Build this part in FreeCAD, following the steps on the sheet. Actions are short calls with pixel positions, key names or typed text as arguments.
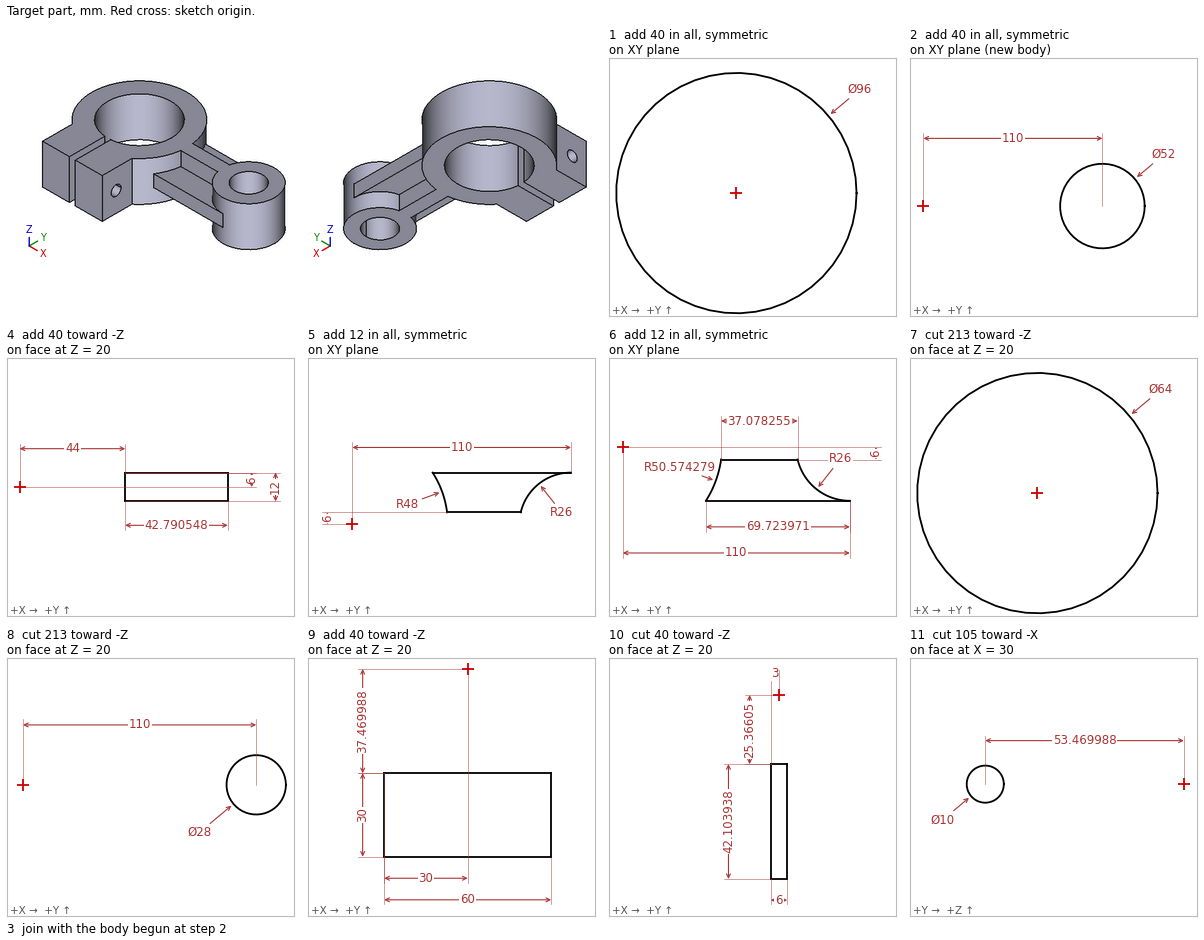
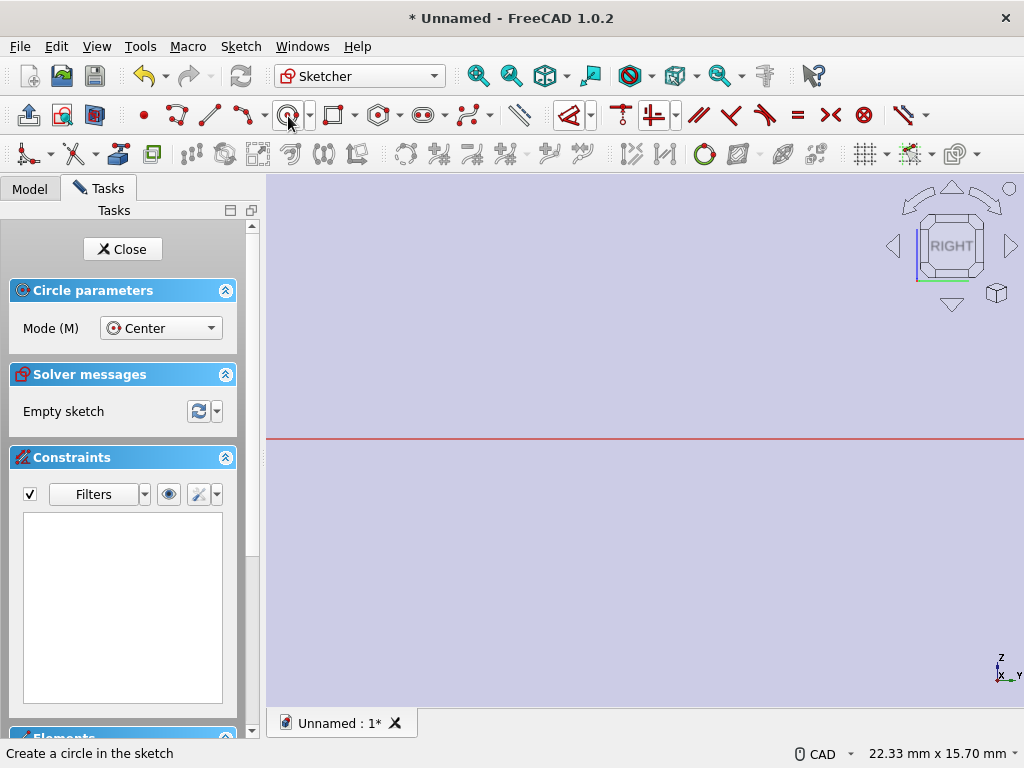
click(570, 439)
click(690, 319)
key(Escape)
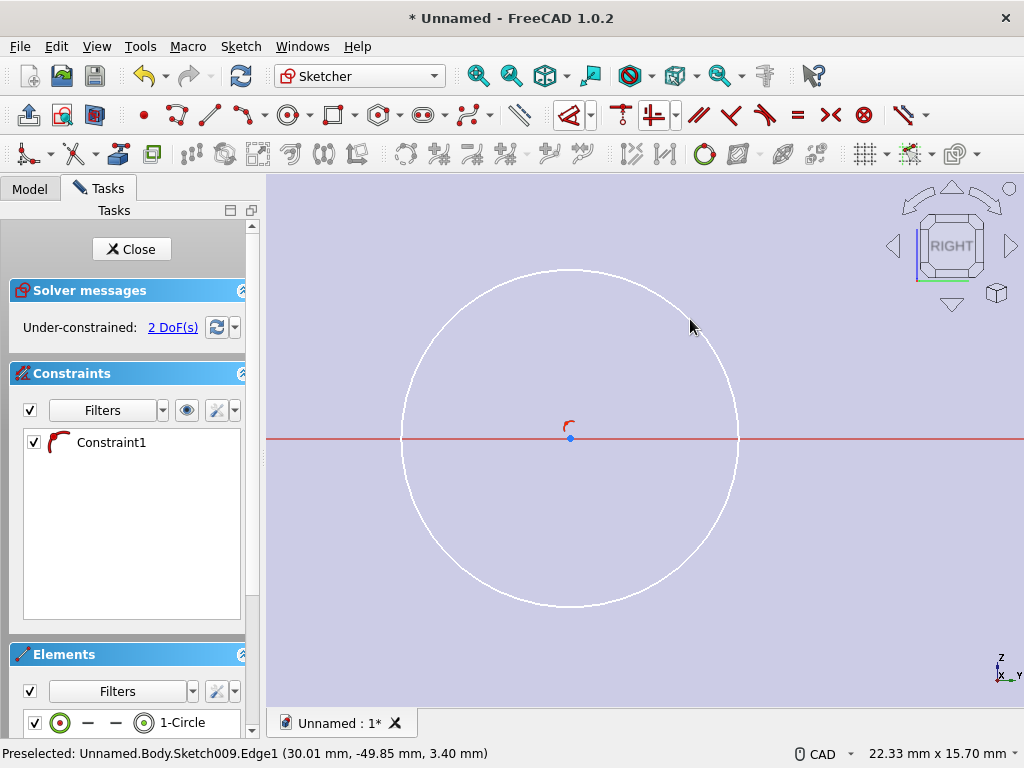
click(689, 319)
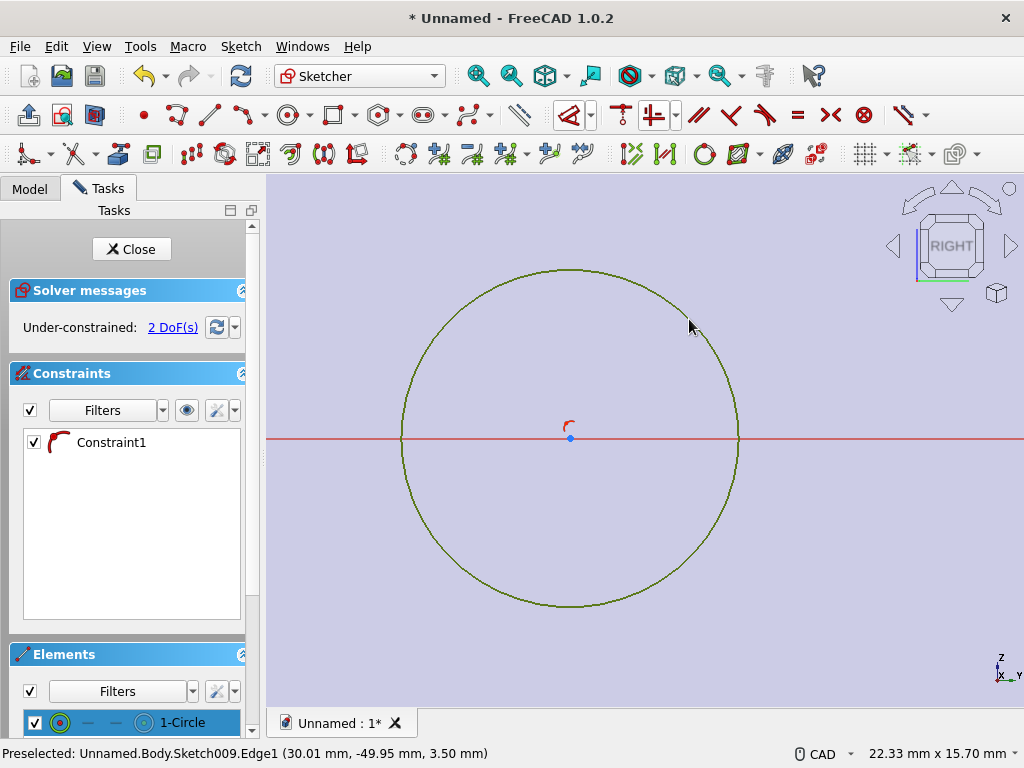
click(590, 116)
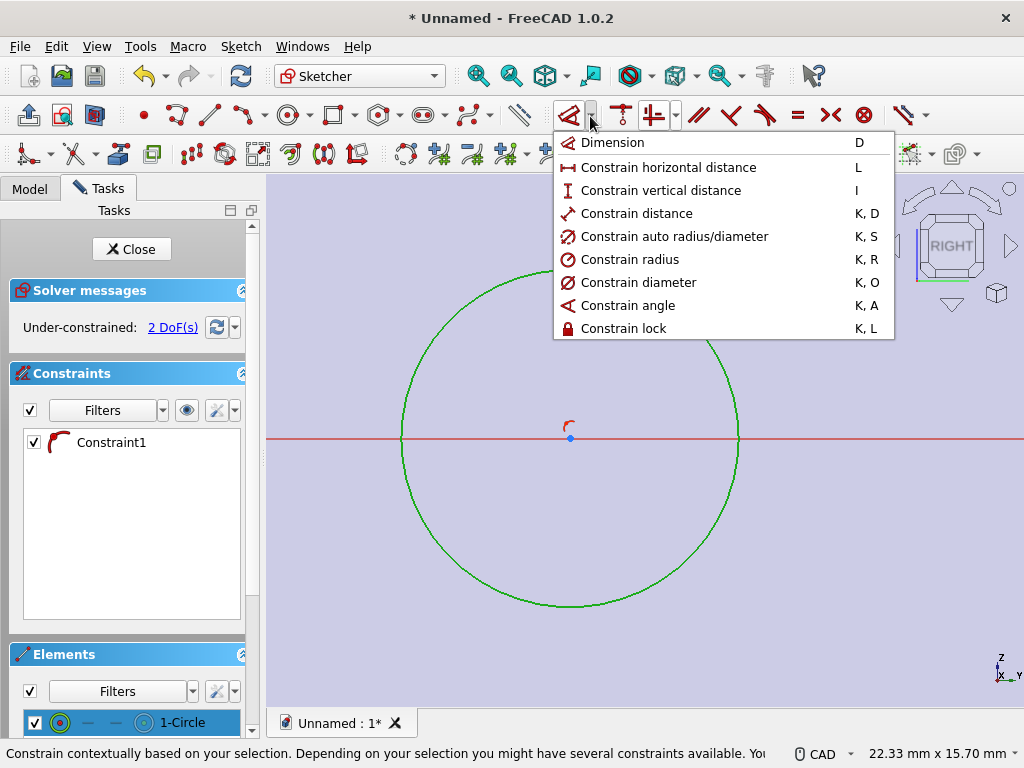
click(724, 282)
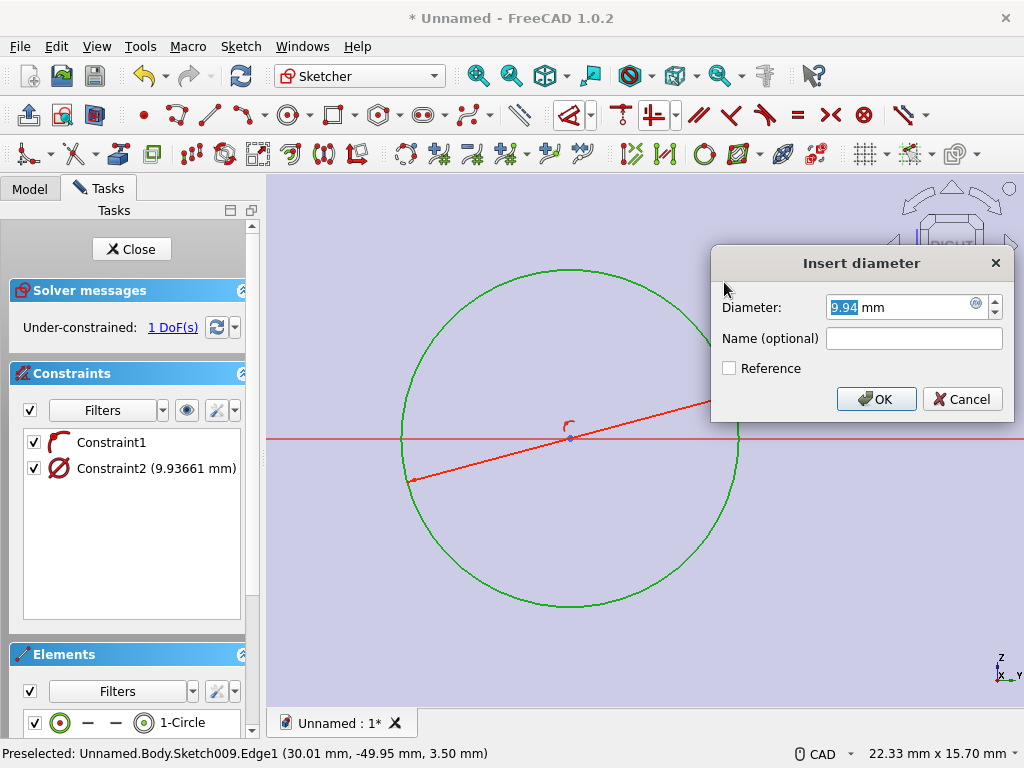
text(10)
key(Return)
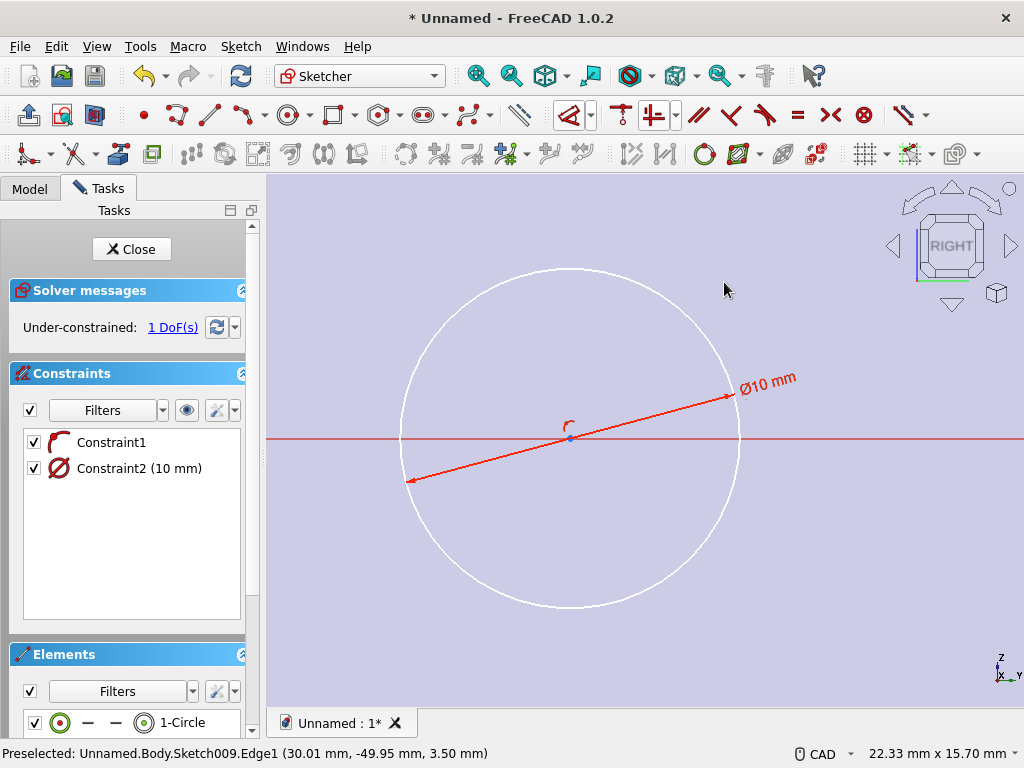
click(570, 439)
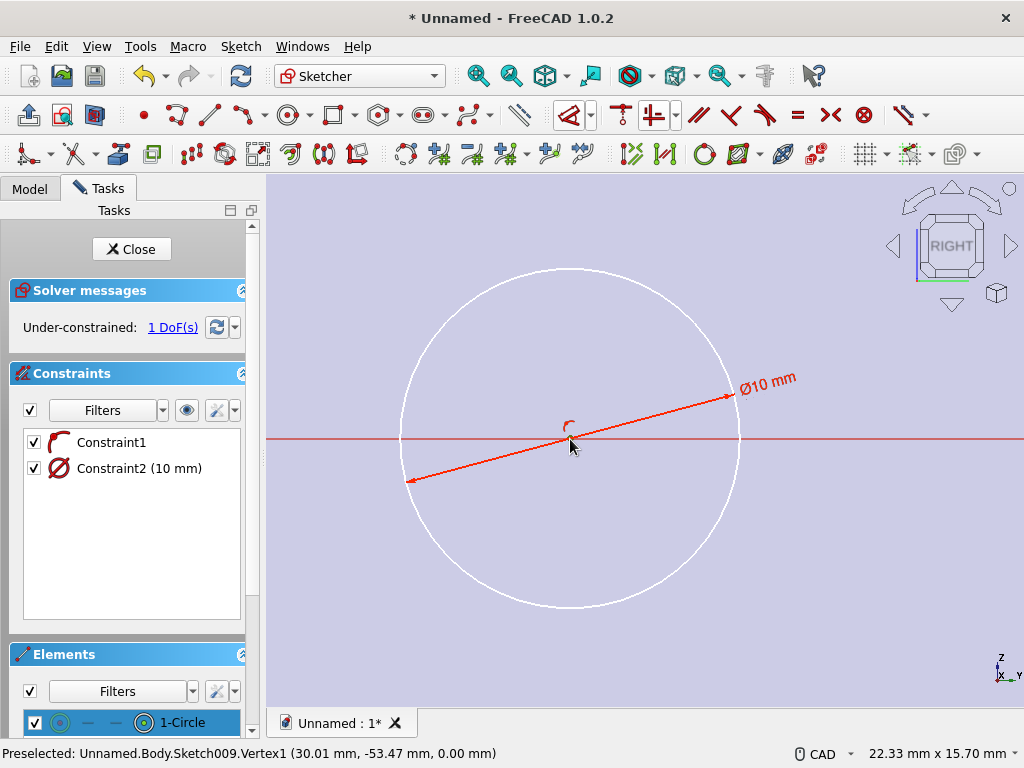
click(590, 116)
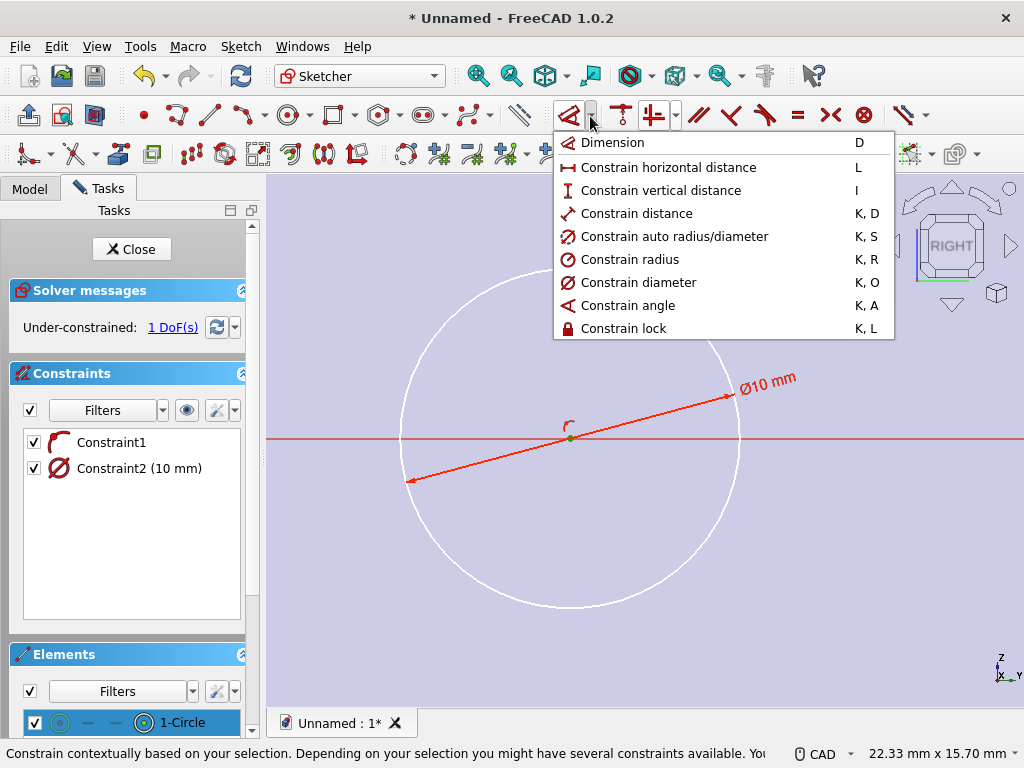
click(724, 168)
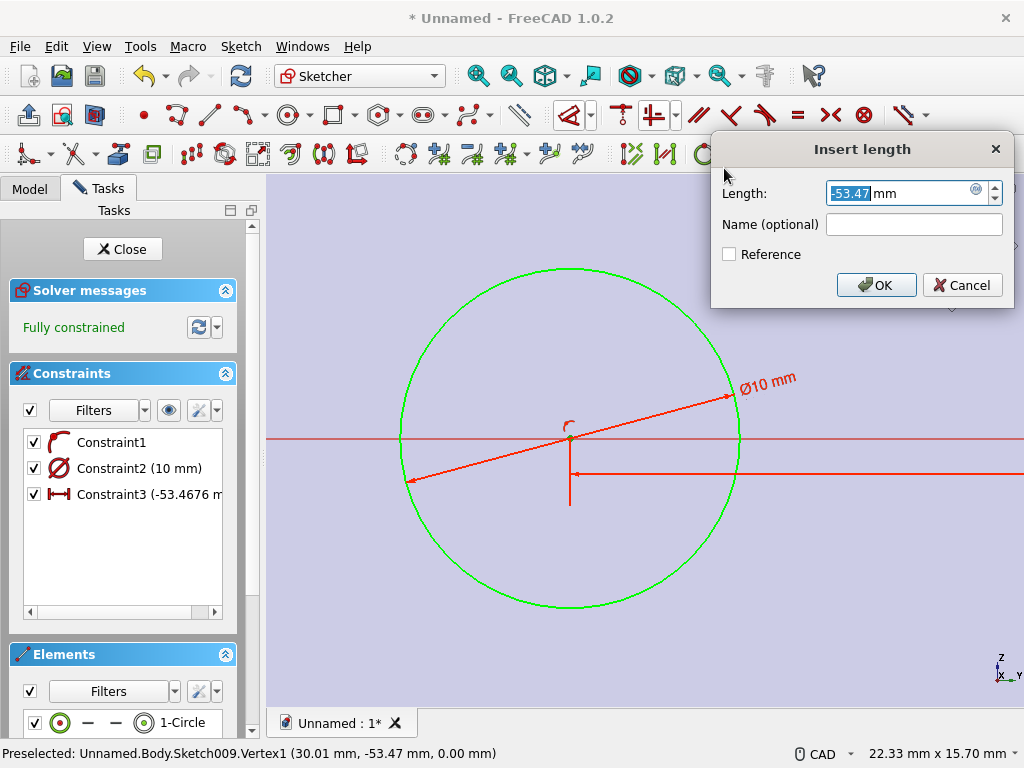
text(-53.469988)
key(Return)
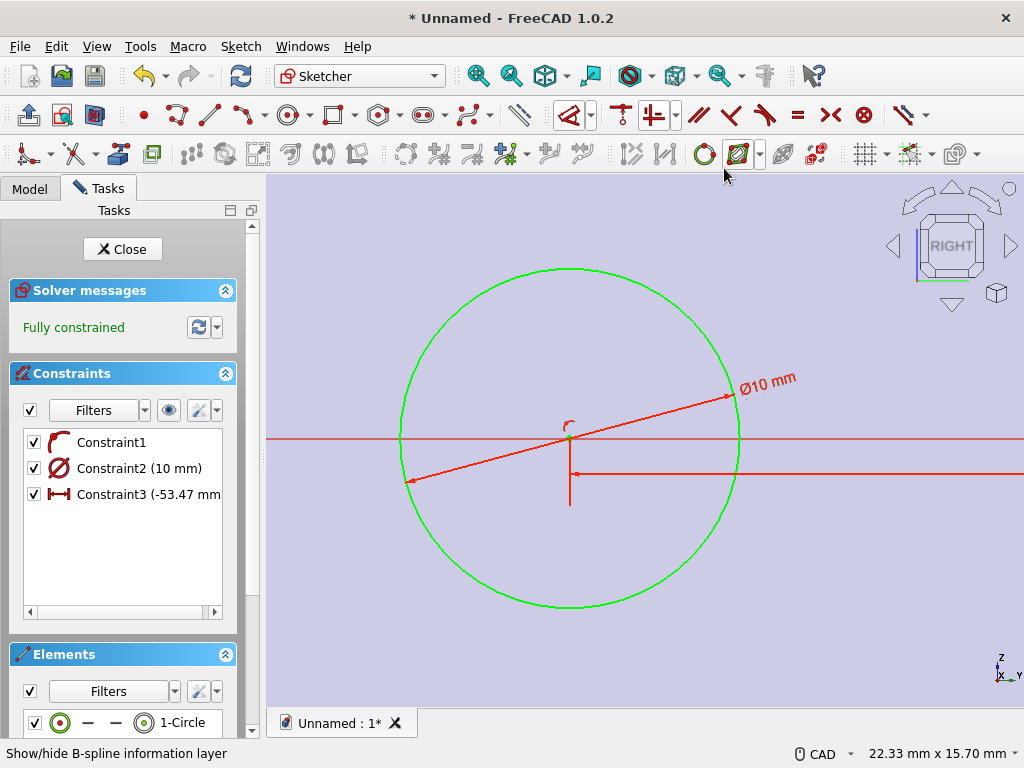
click(123, 249)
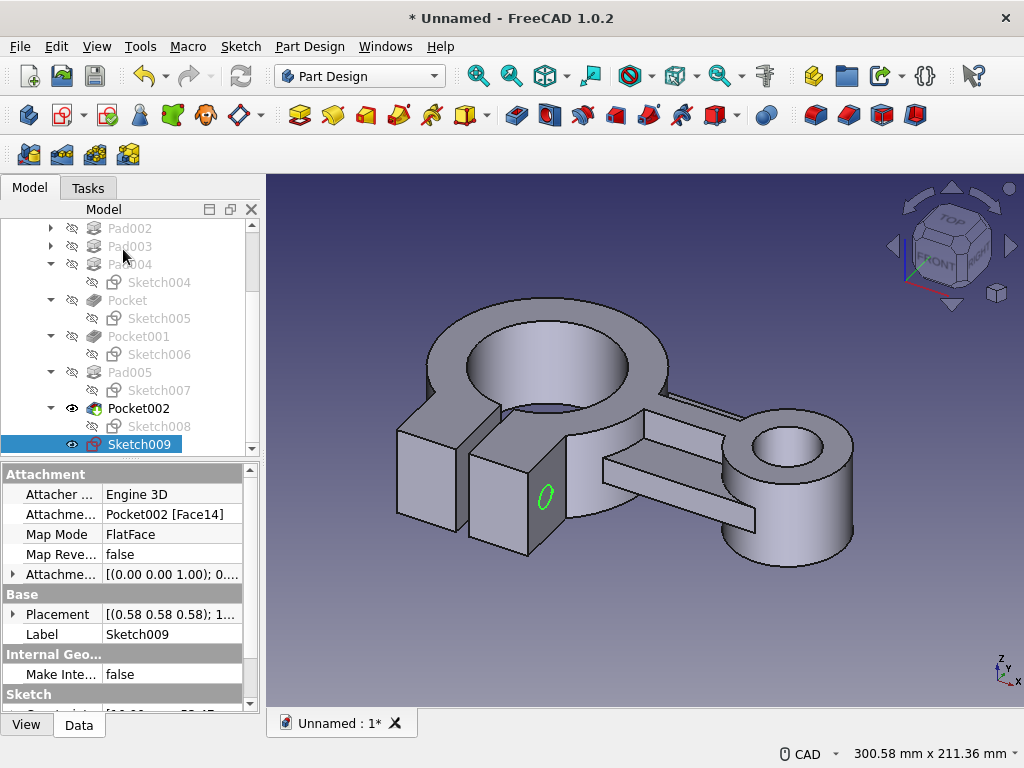
click(517, 116)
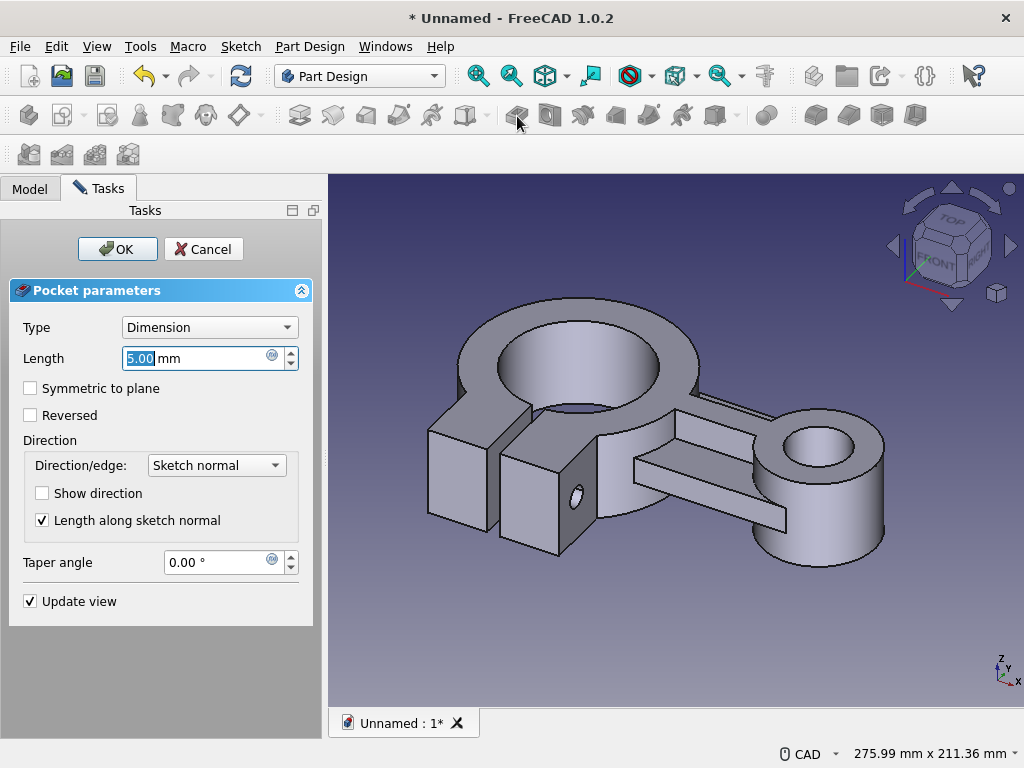
text(105)
key(Tab)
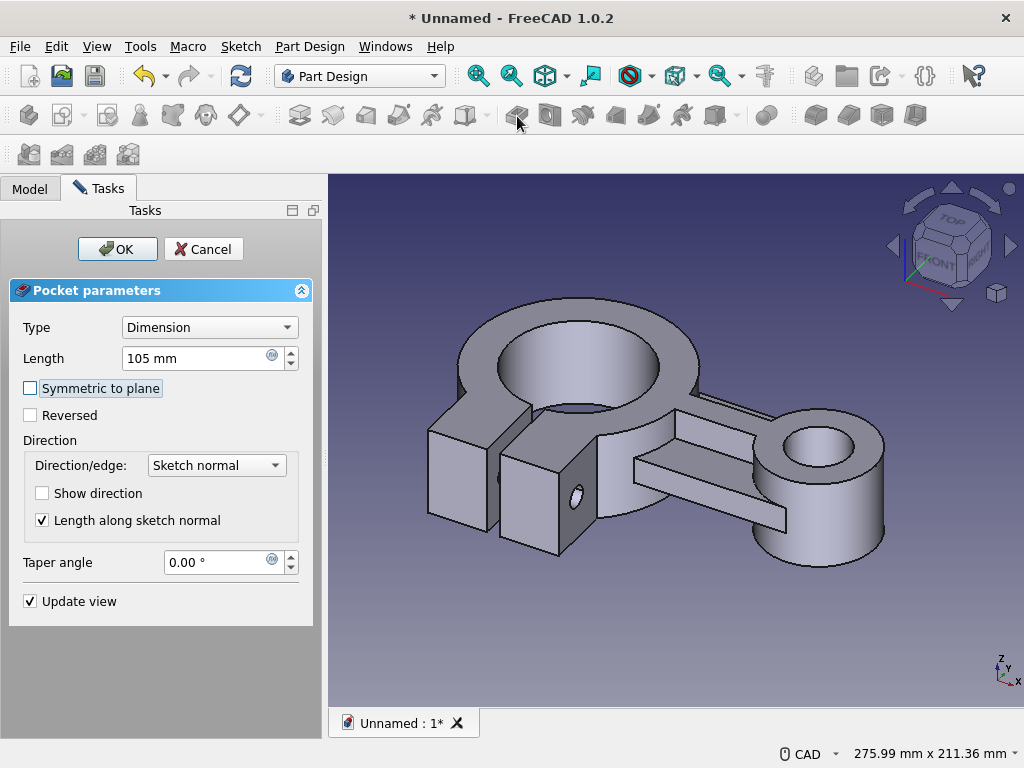
click(118, 249)